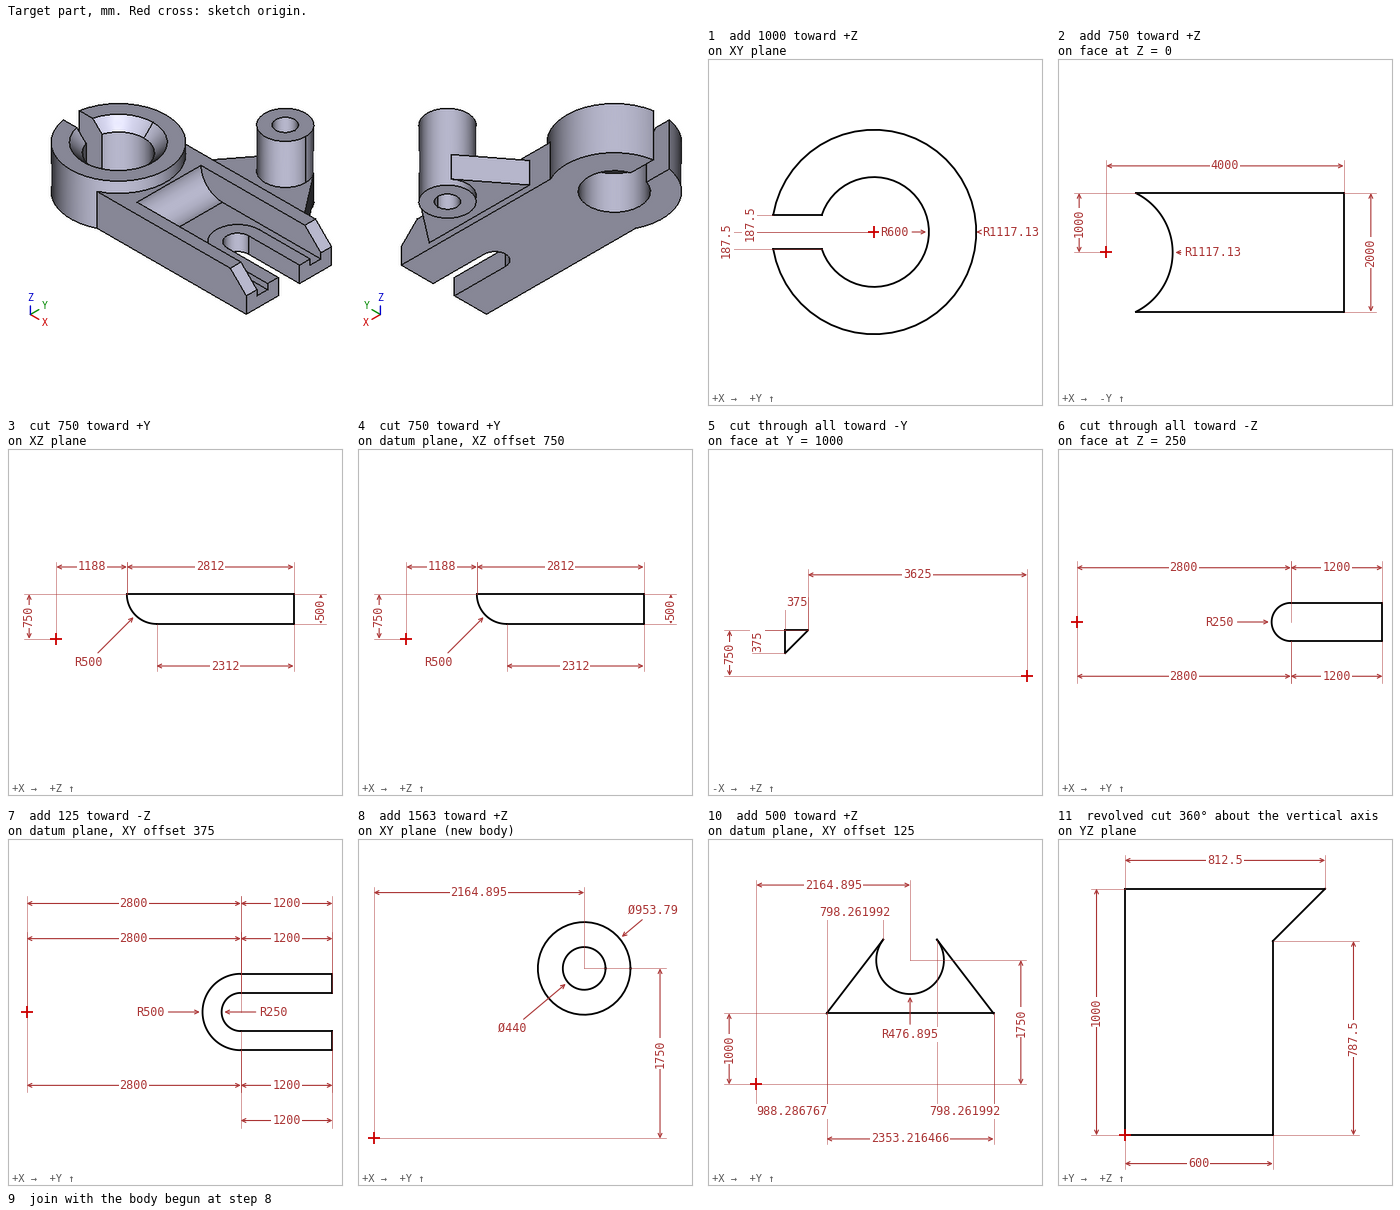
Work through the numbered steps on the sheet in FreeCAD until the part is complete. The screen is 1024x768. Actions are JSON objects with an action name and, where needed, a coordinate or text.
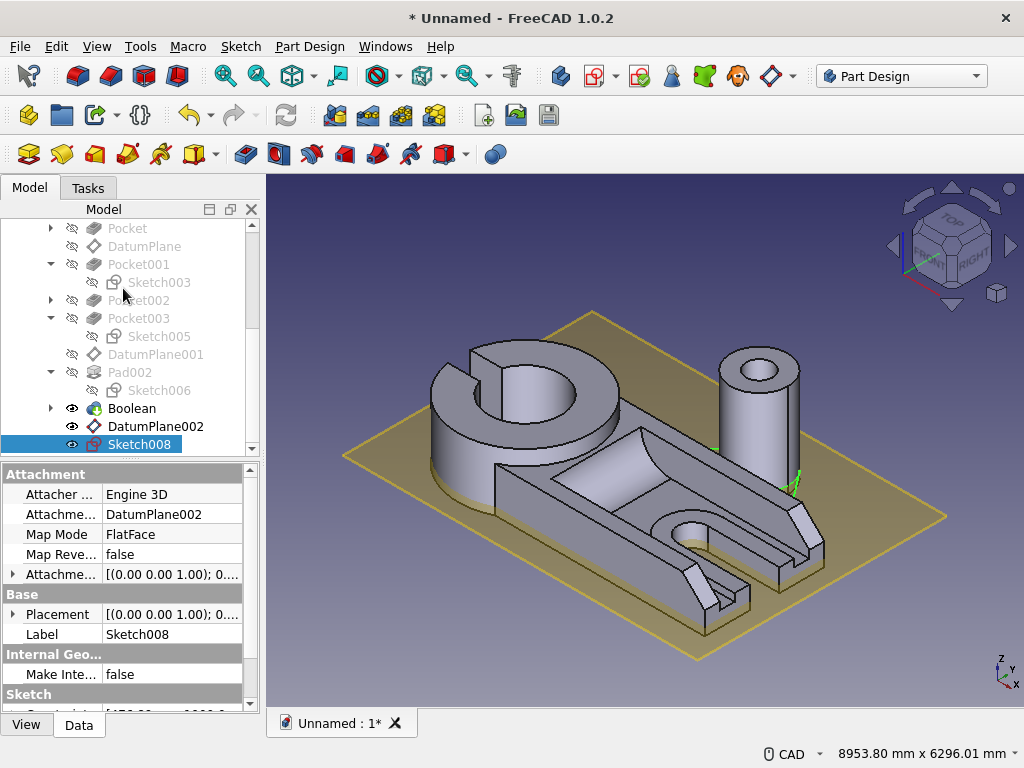
{"action": "left_click", "coordinate": [29, 154]}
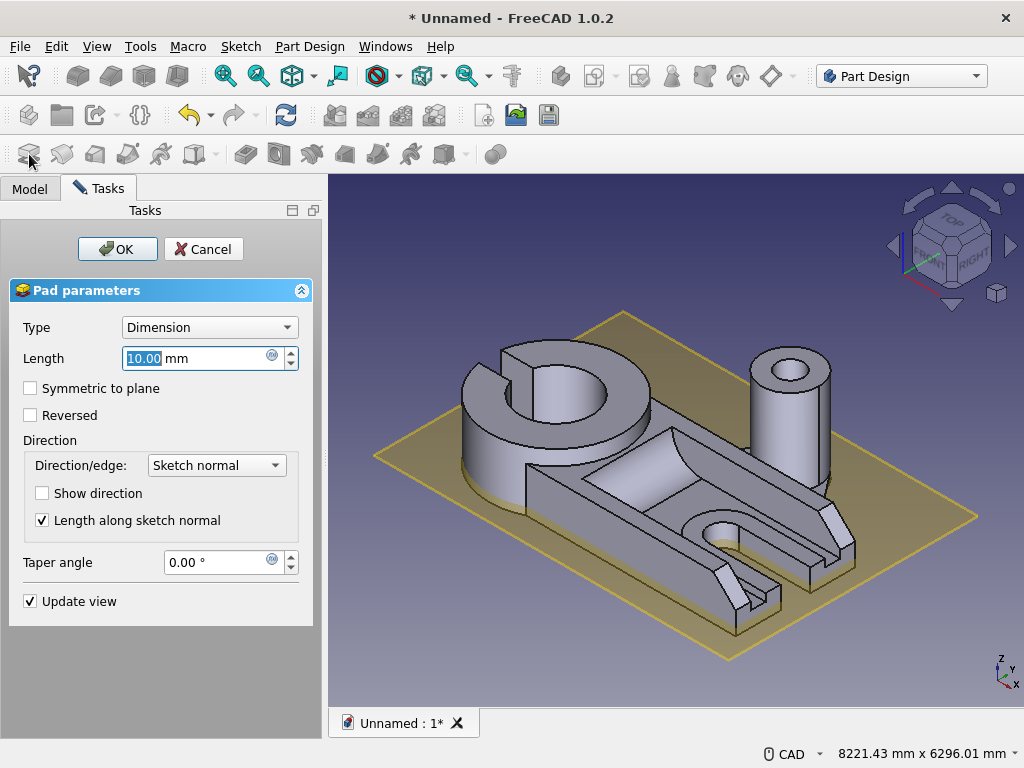
{"action": "type", "text": "500"}
{"action": "key", "text": "Tab"}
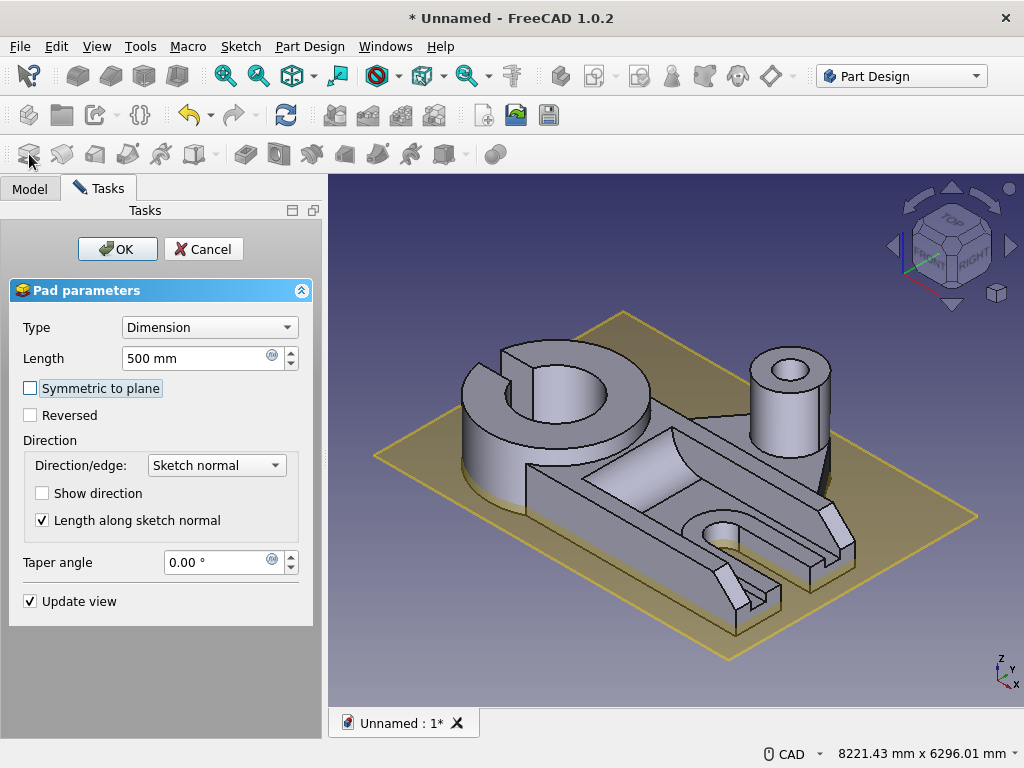
{"action": "left_click", "coordinate": [118, 249]}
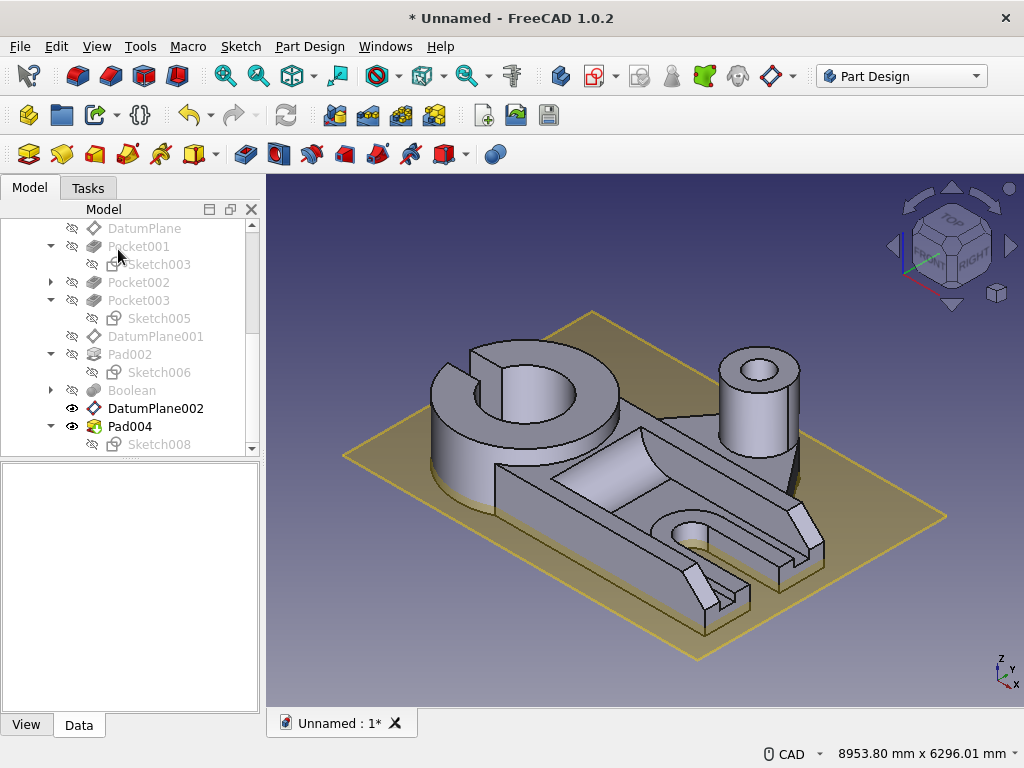
{"action": "left_click", "coordinate": [117, 408]}
{"action": "key", "text": "space"}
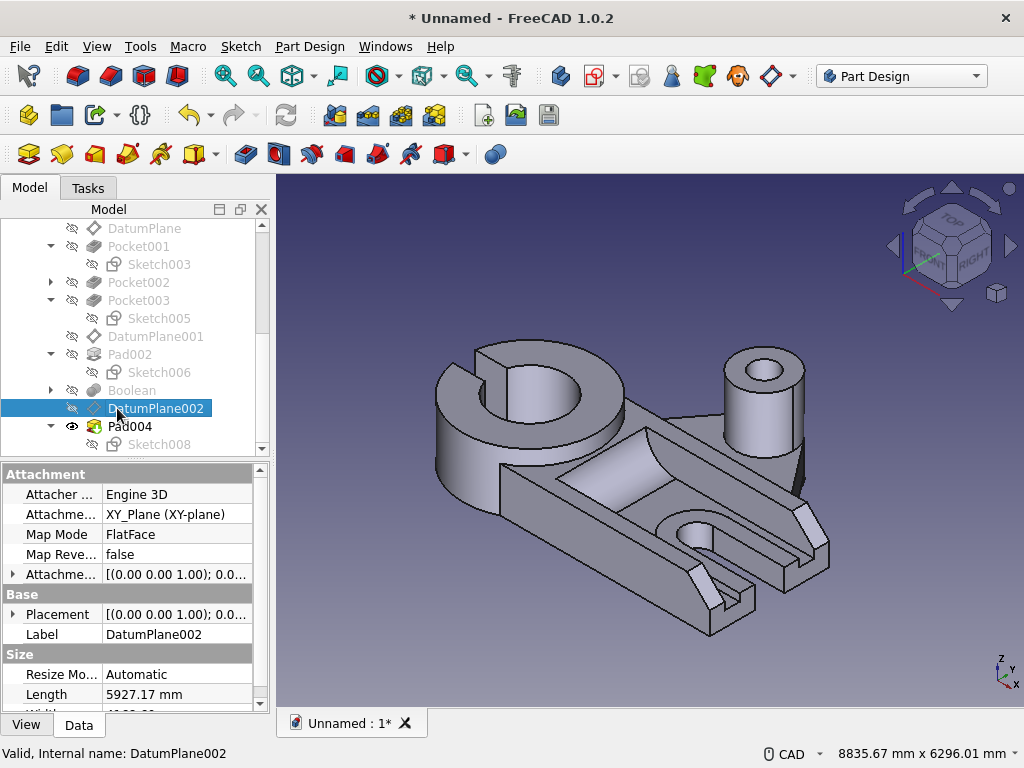
{"action": "left_click", "coordinate": [316, 667]}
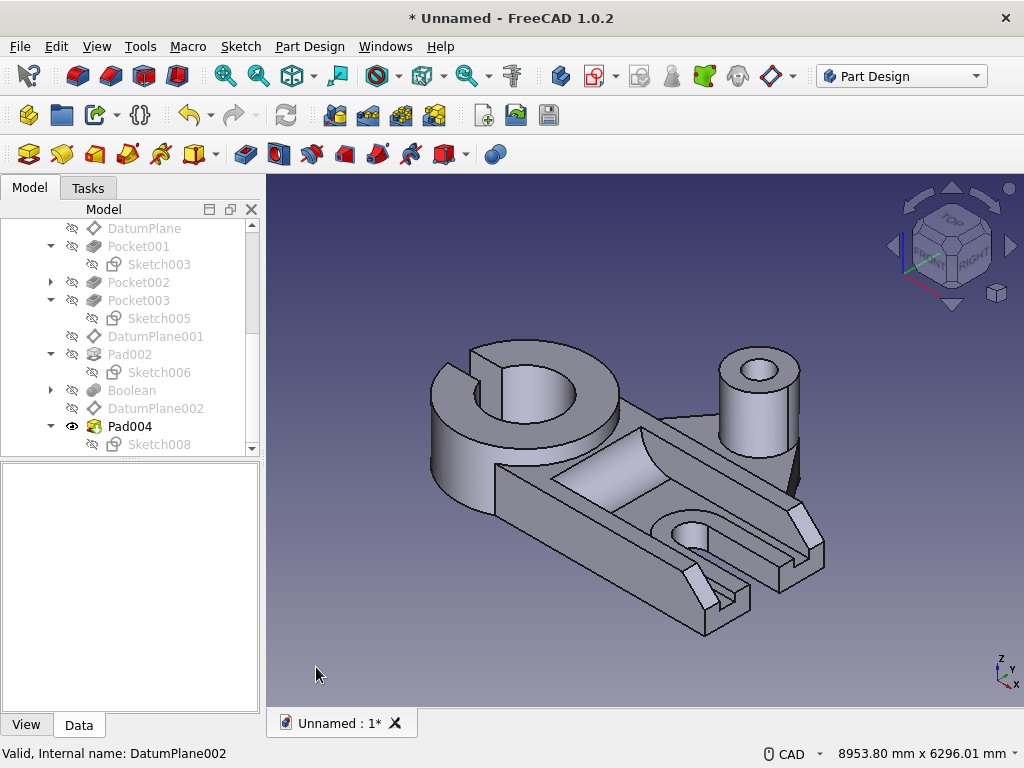
{"action": "left_click", "coordinate": [594, 76]}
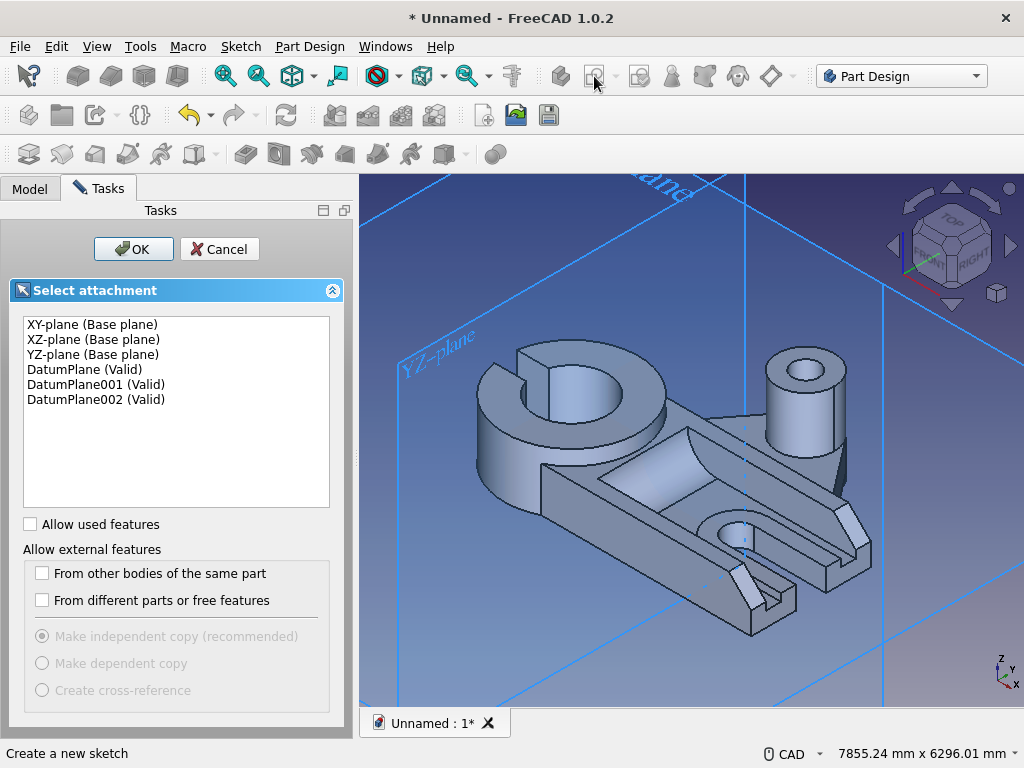
{"action": "left_click", "coordinate": [84, 354]}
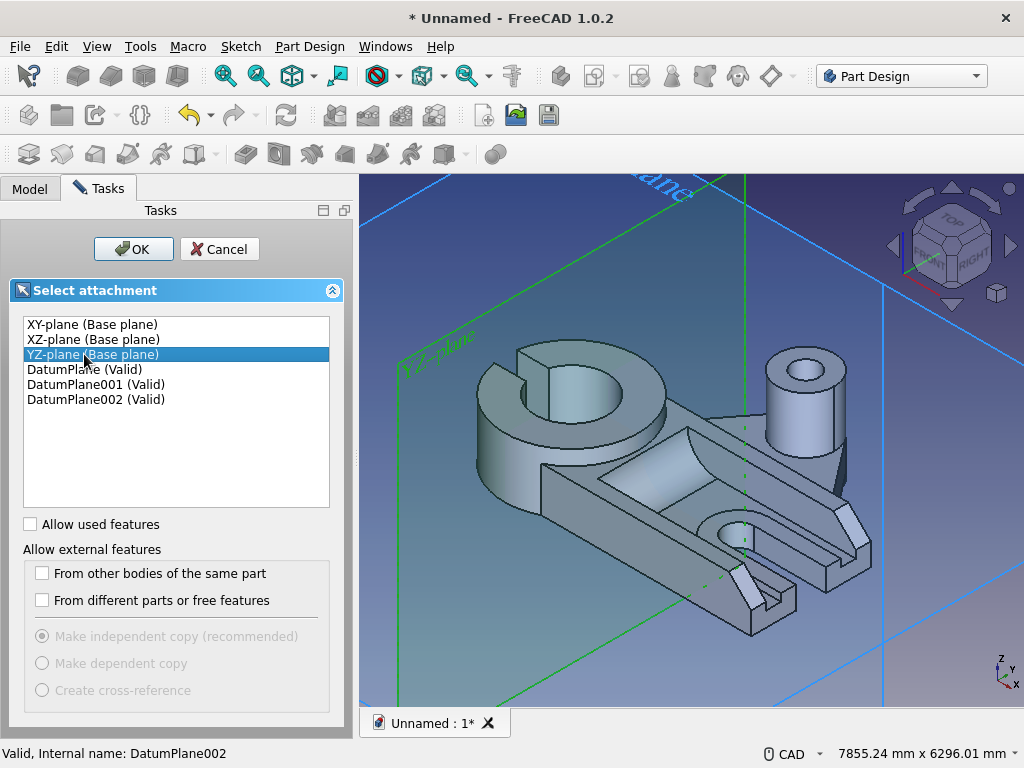
{"action": "left_click", "coordinate": [134, 249]}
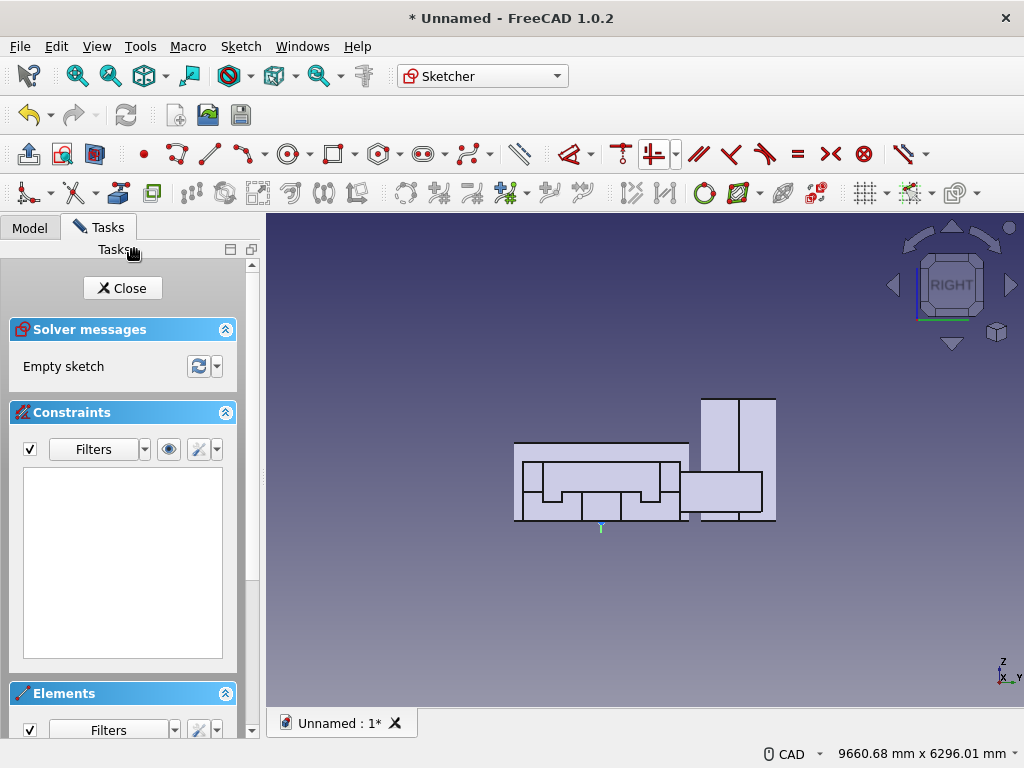
{"action": "left_click", "coordinate": [95, 154]}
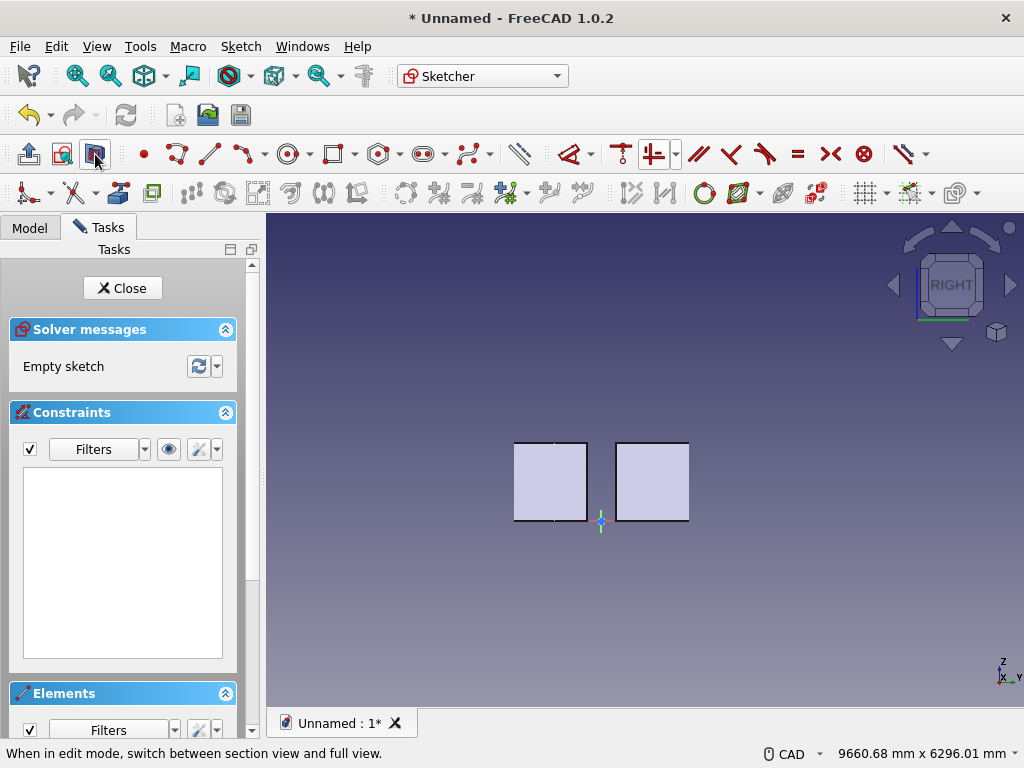
{"action": "scroll", "coordinate": [652, 489], "scroll_direction": "up", "scroll_amount": 7}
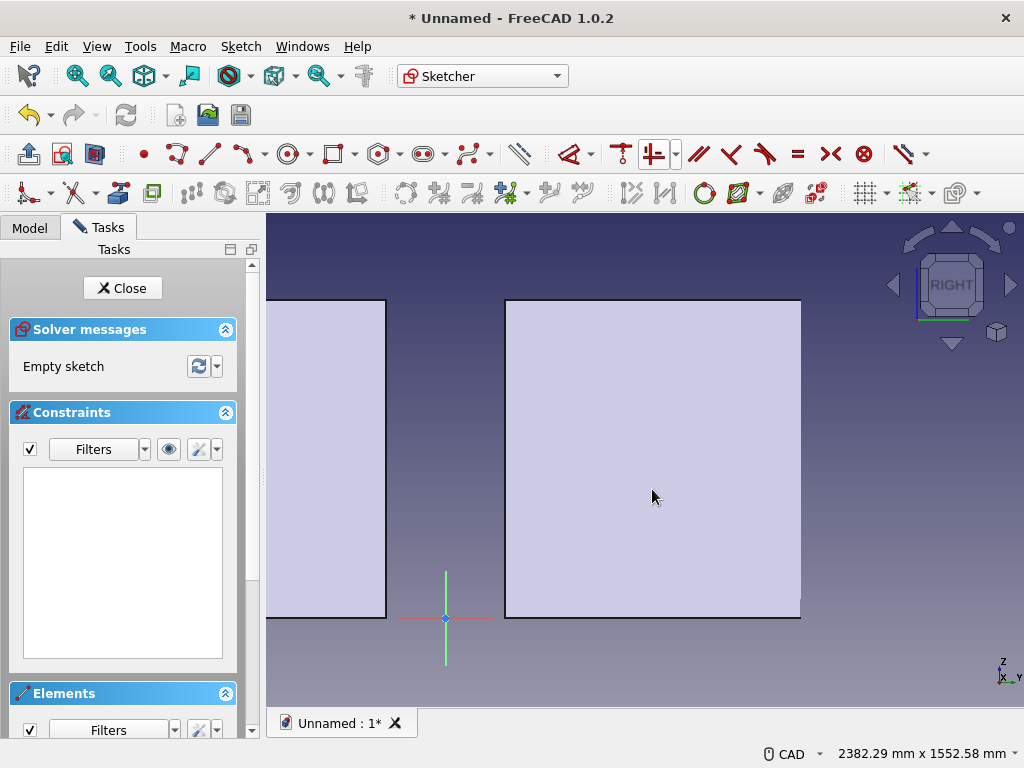
{"action": "key", "text": "g m"}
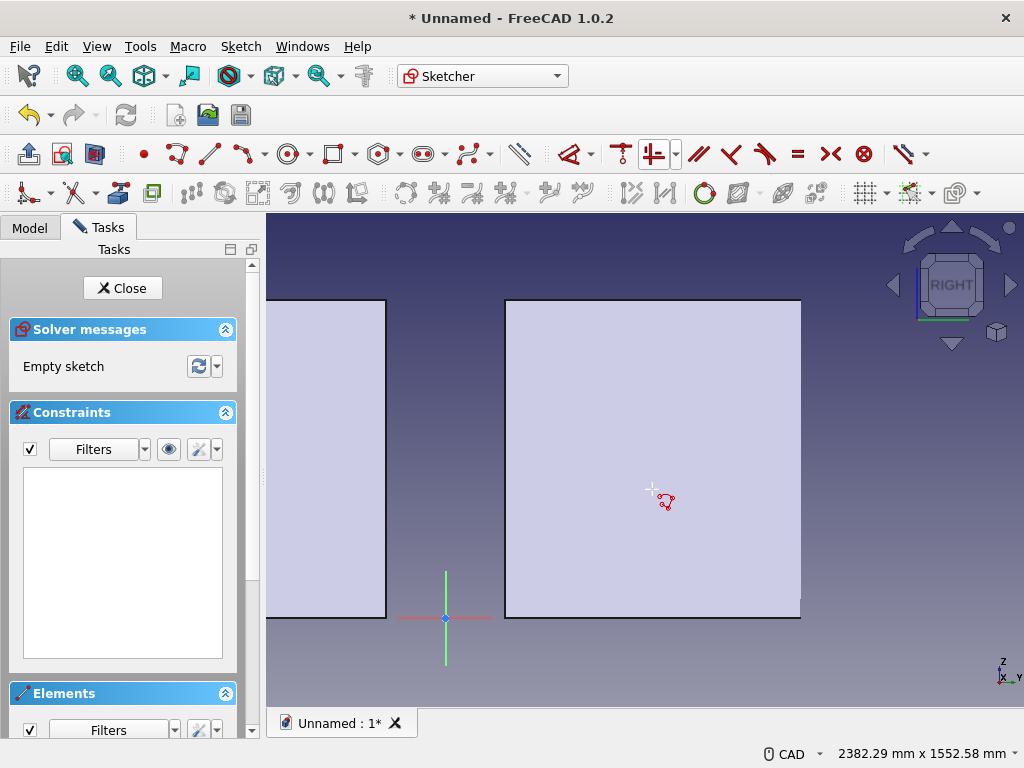
{"action": "left_click", "coordinate": [446, 618]}
{"action": "left_click", "coordinate": [637, 609]}
{"action": "left_click", "coordinate": [637, 368]}
{"action": "left_click", "coordinate": [704, 300]}
{"action": "left_click", "coordinate": [455, 300]}
{"action": "left_click", "coordinate": [446, 618]}
{"action": "key", "text": "Escape"}
{"action": "key", "text": "Escape"}